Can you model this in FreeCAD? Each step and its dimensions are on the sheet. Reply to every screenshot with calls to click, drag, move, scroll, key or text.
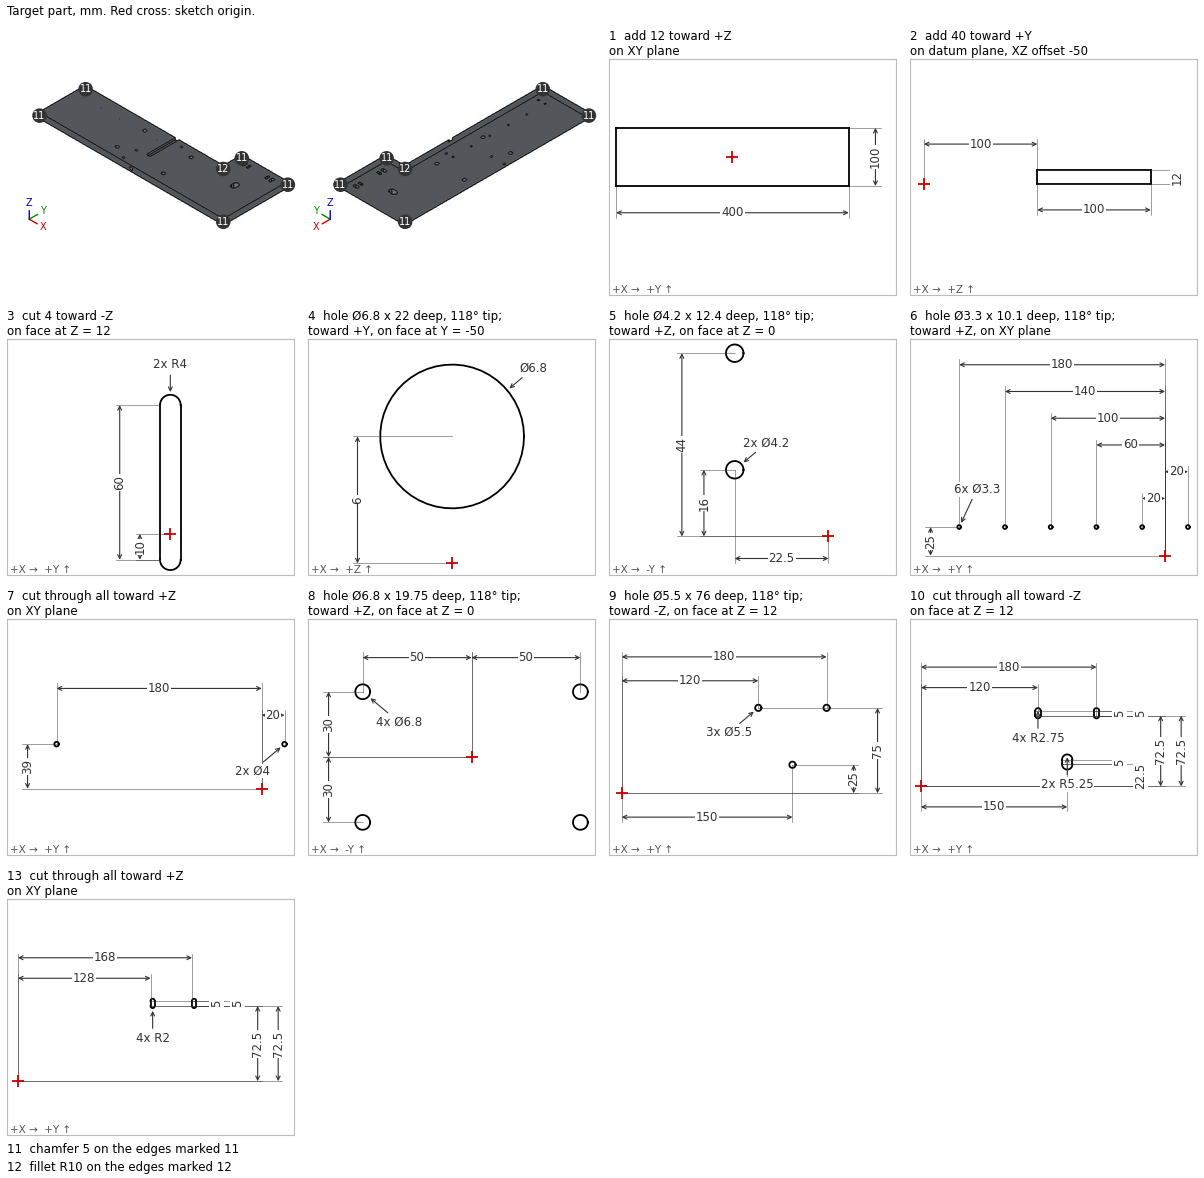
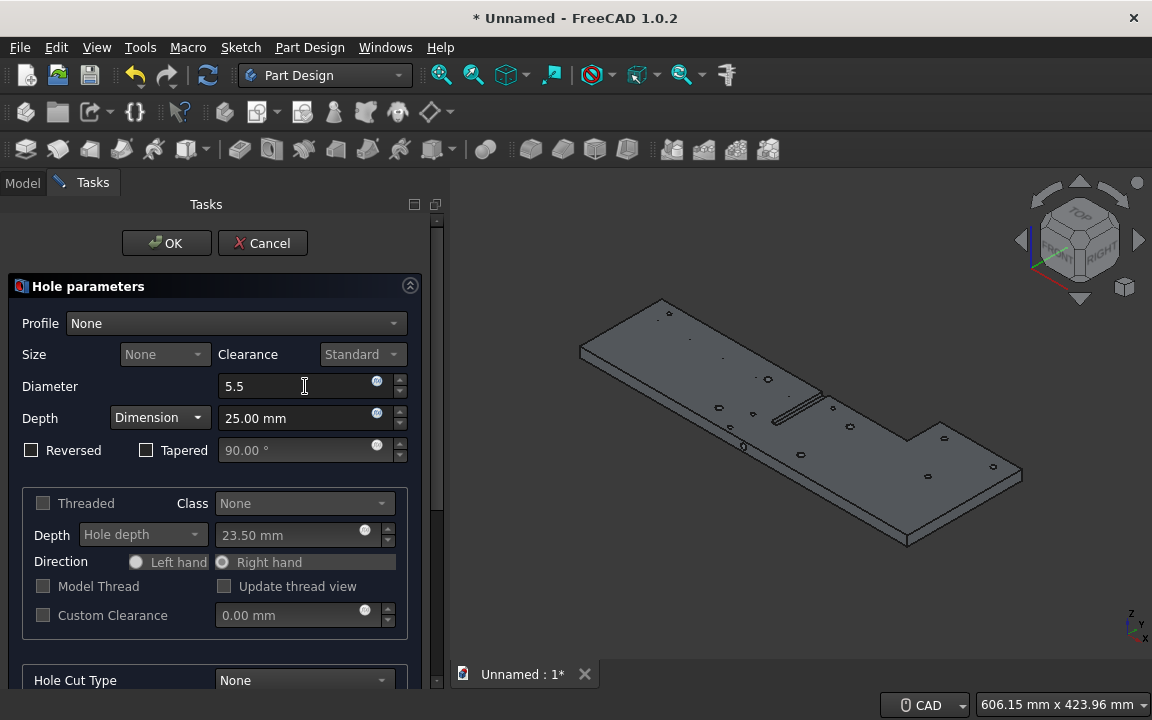
triple_click(305, 418)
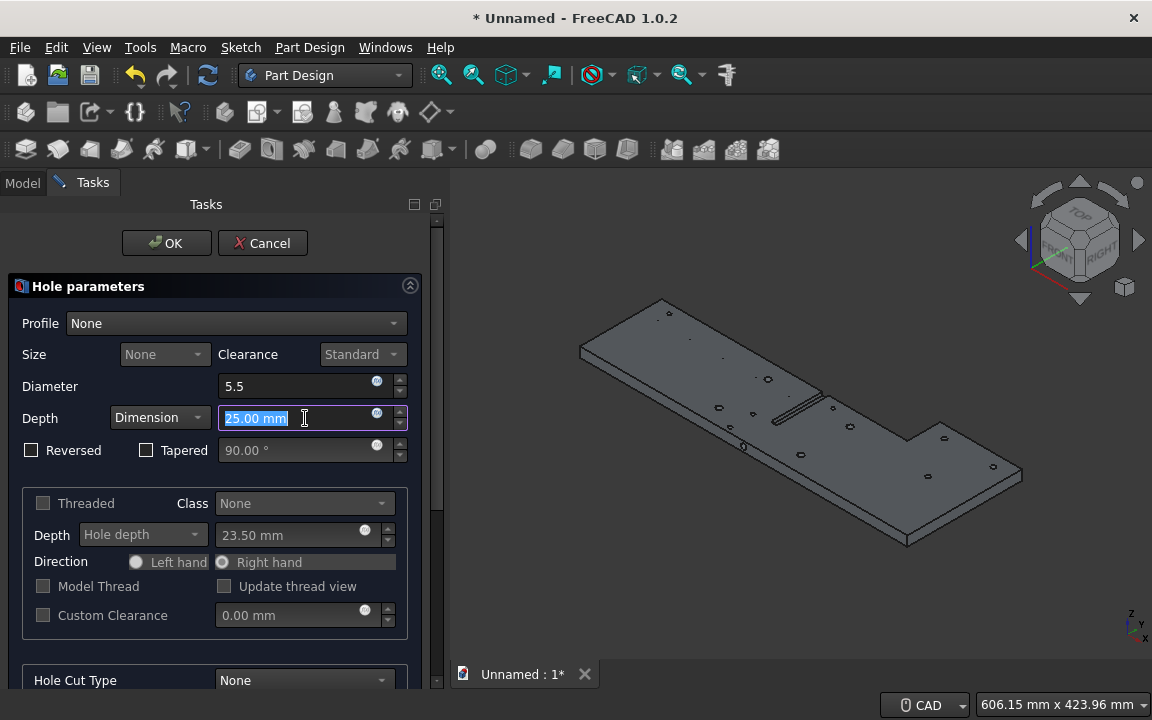
text(76)
key(Tab)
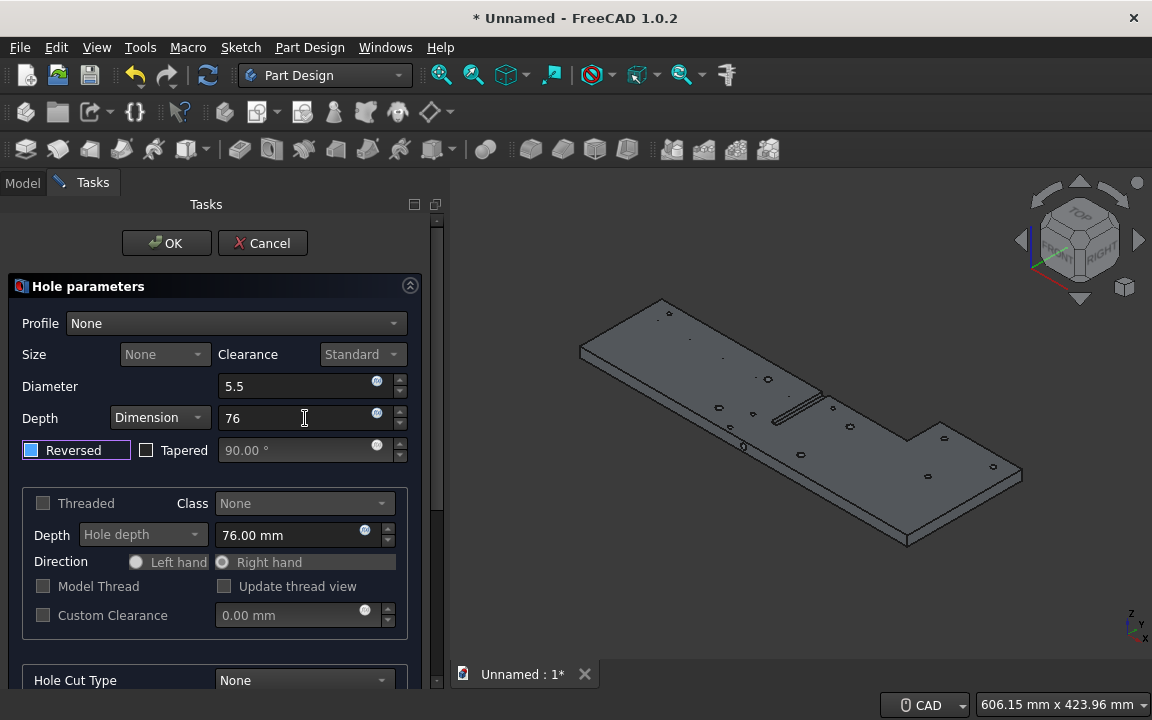
click(167, 243)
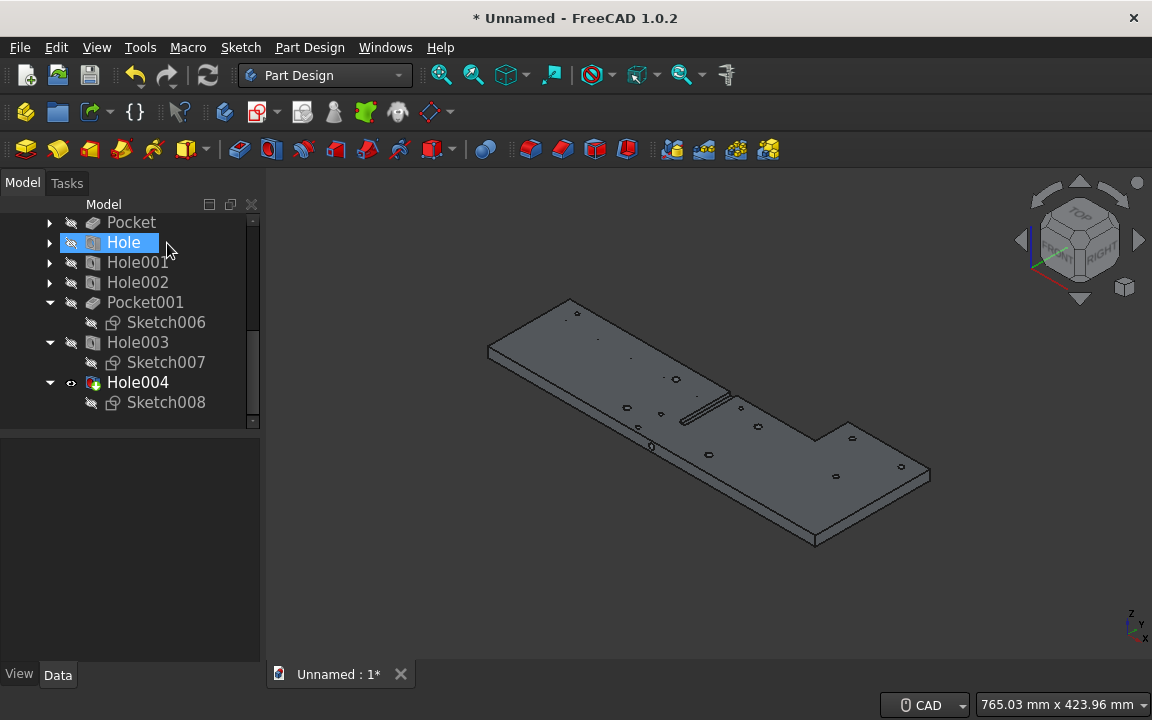
click(599, 362)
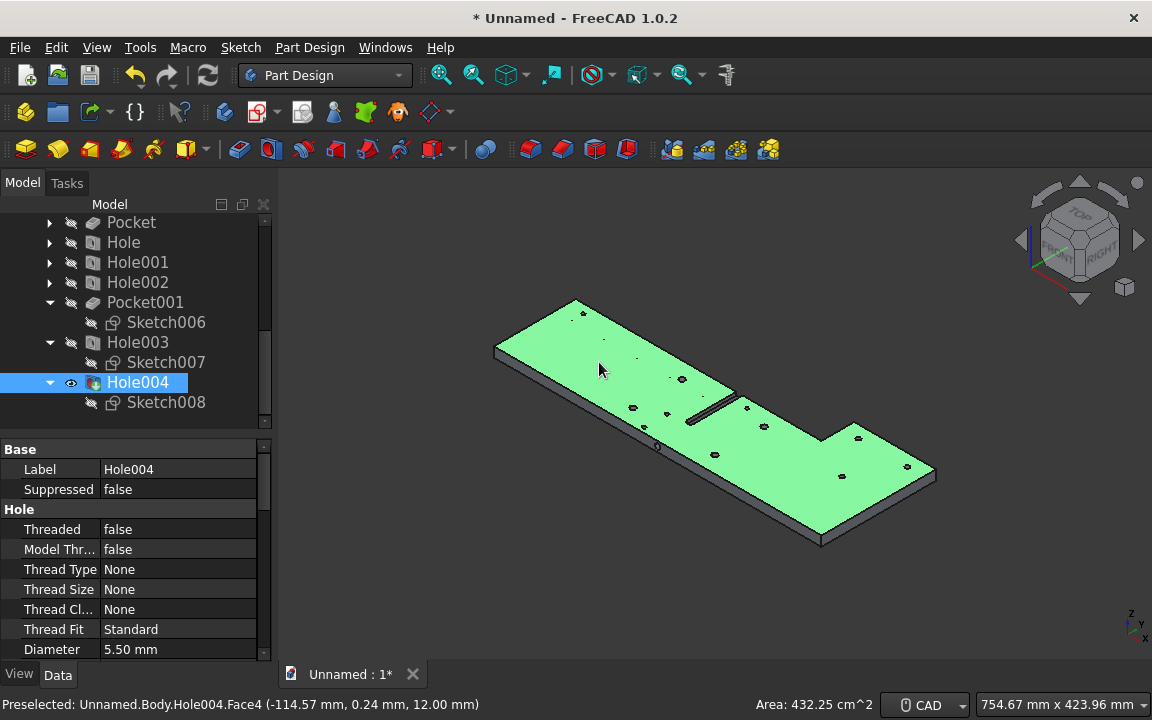
click(258, 112)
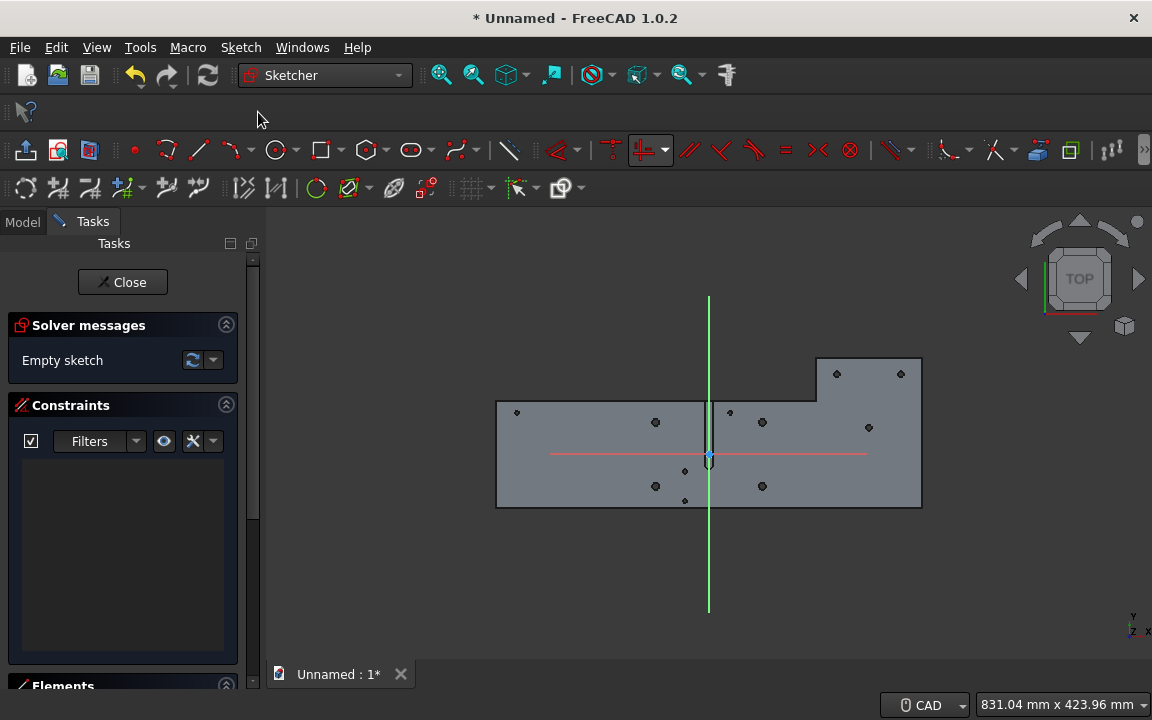
scroll(944, 392, up, 7)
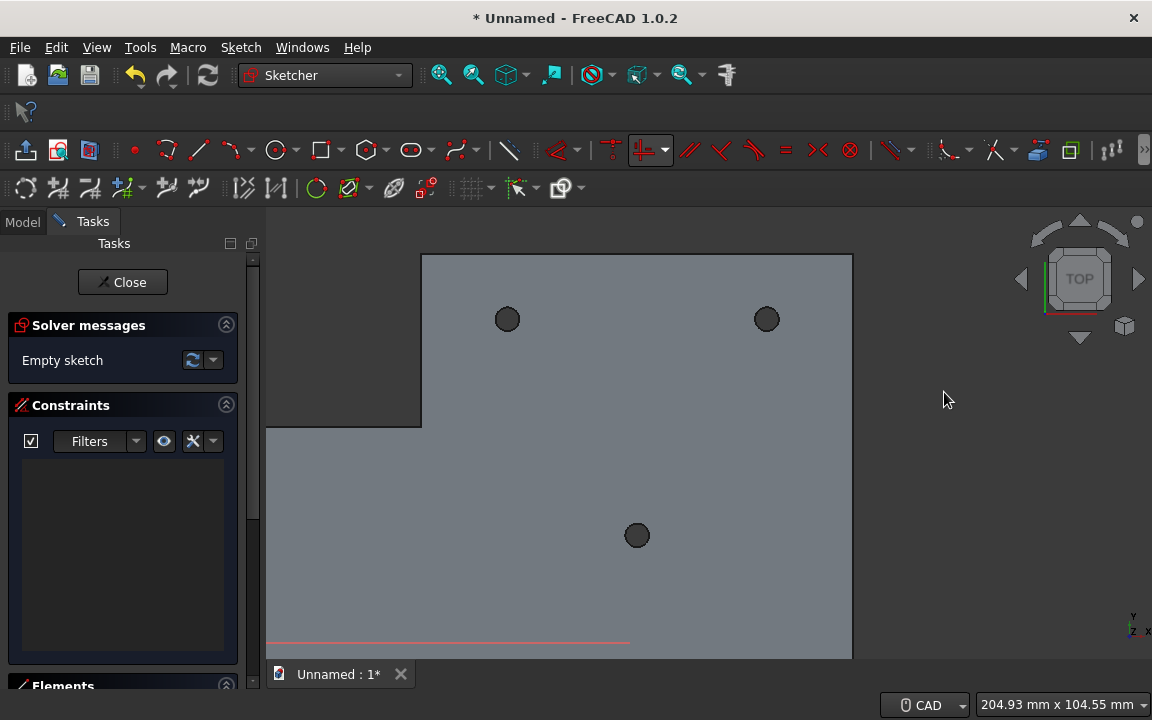
click(412, 150)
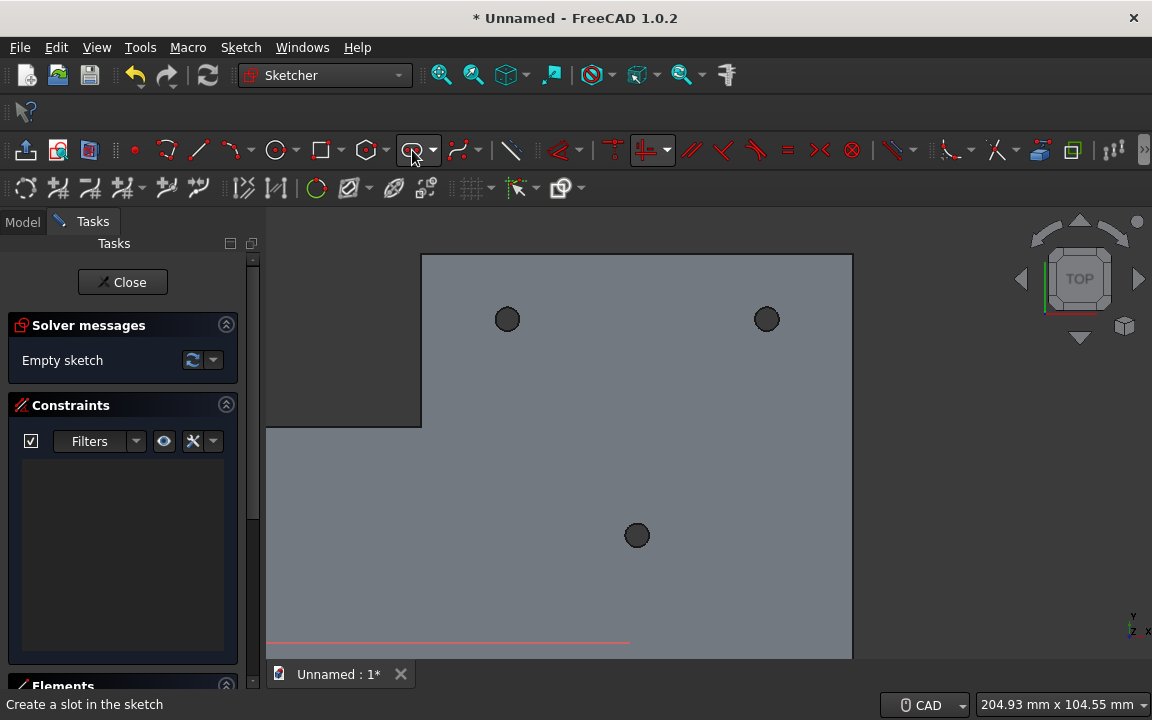
scroll(507, 330, up, 4)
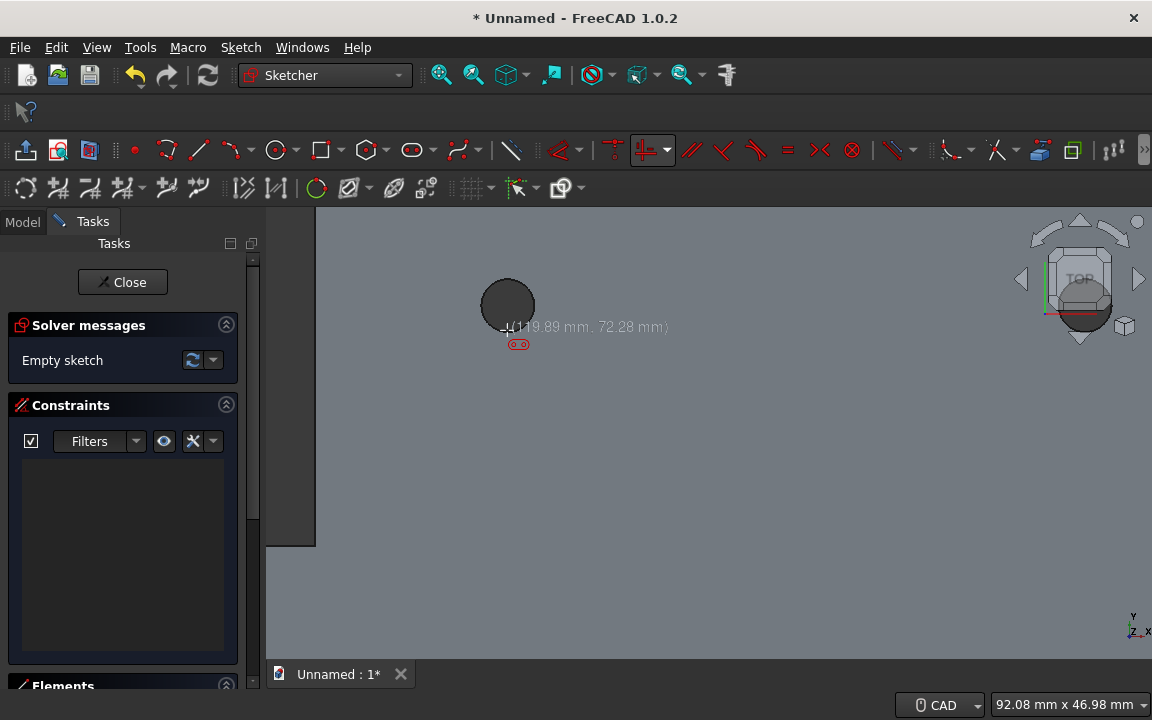
click(508, 330)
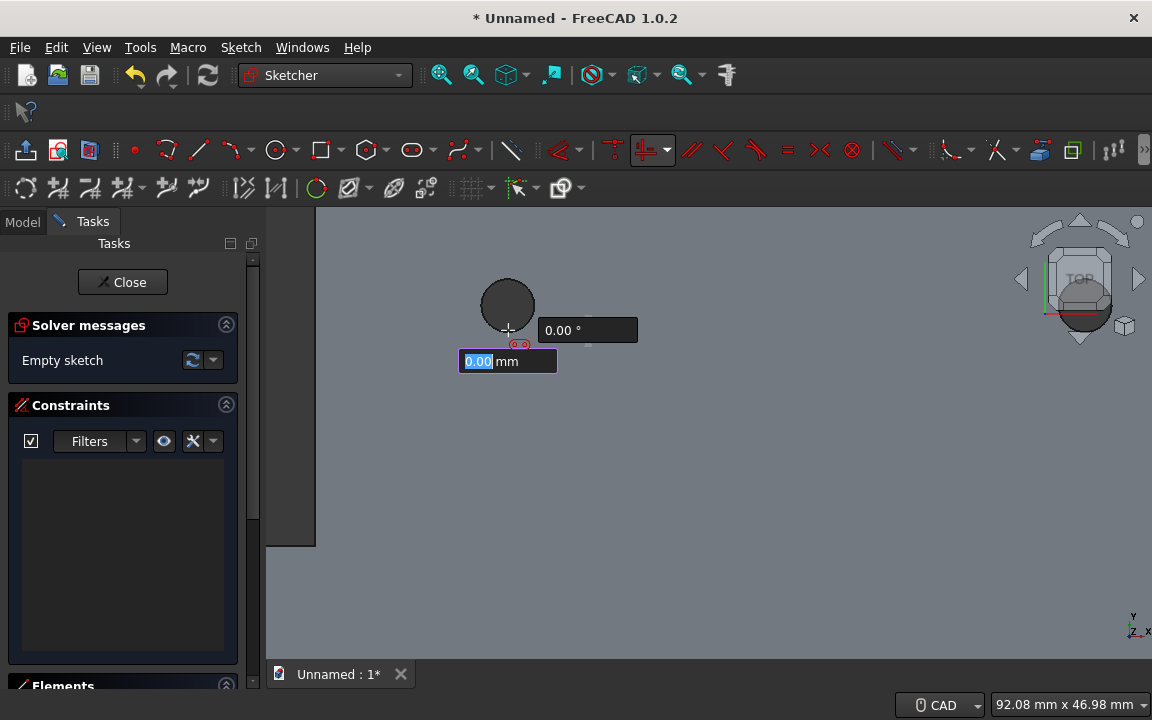
click(508, 282)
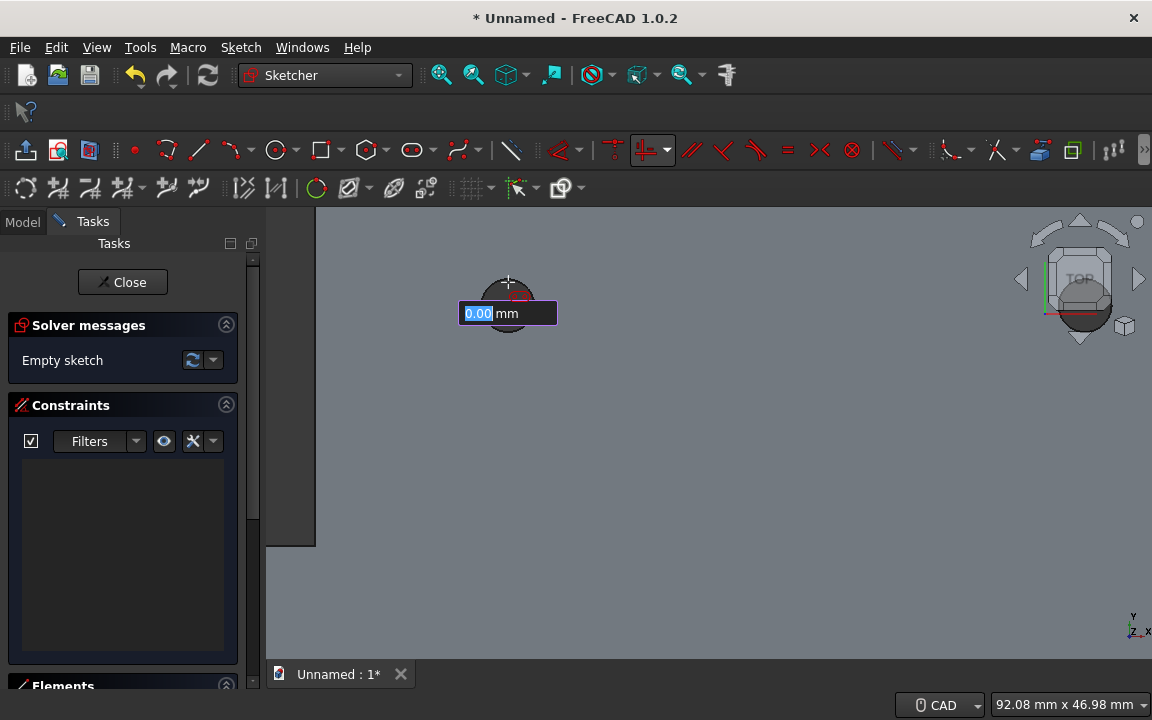
click(534, 306)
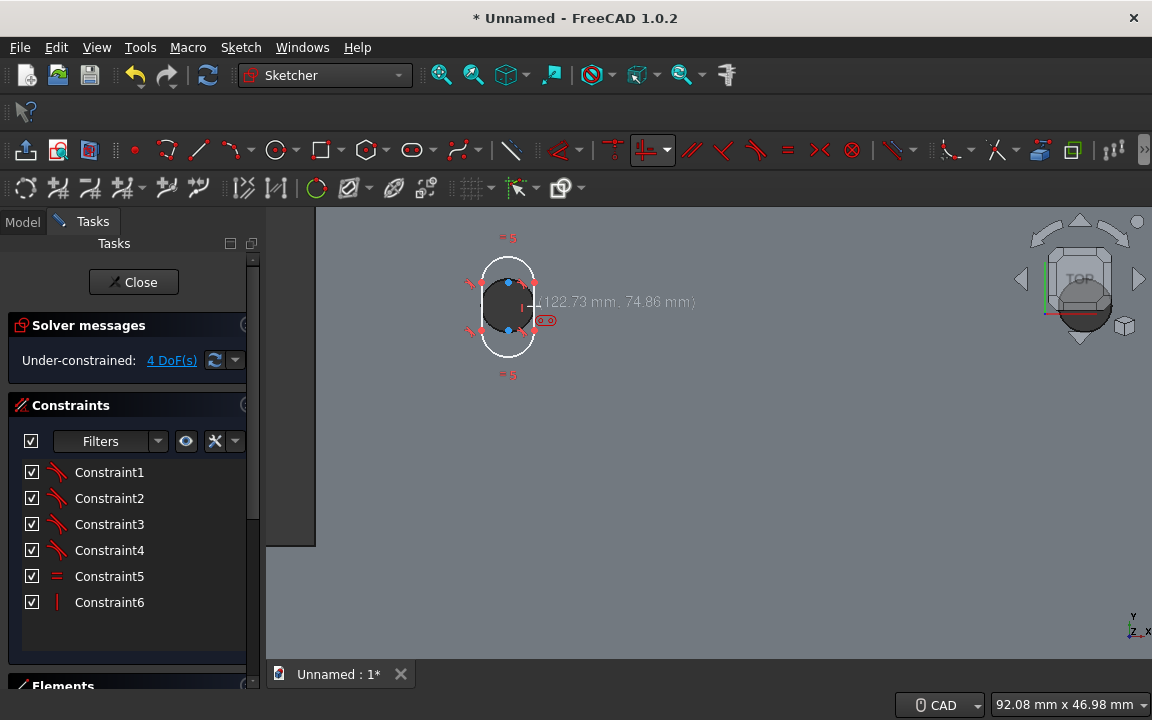
scroll(513, 331, down, 4)